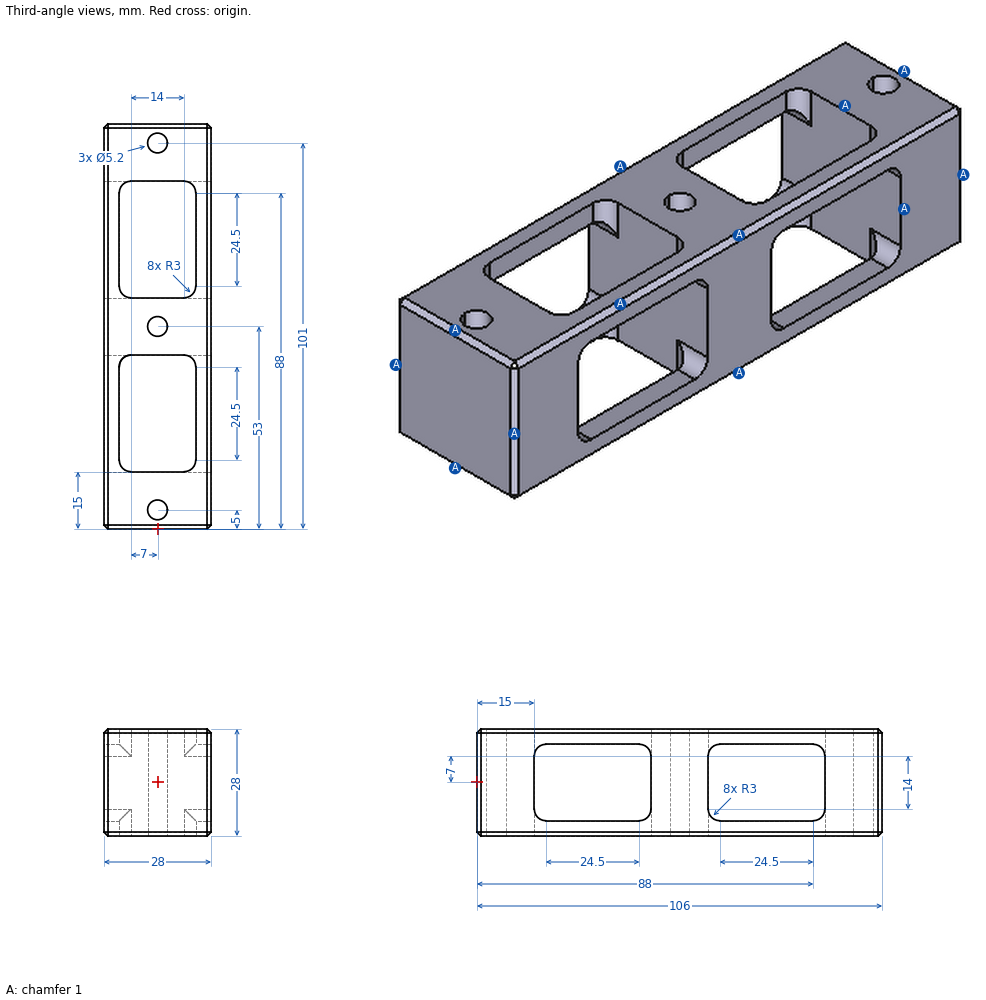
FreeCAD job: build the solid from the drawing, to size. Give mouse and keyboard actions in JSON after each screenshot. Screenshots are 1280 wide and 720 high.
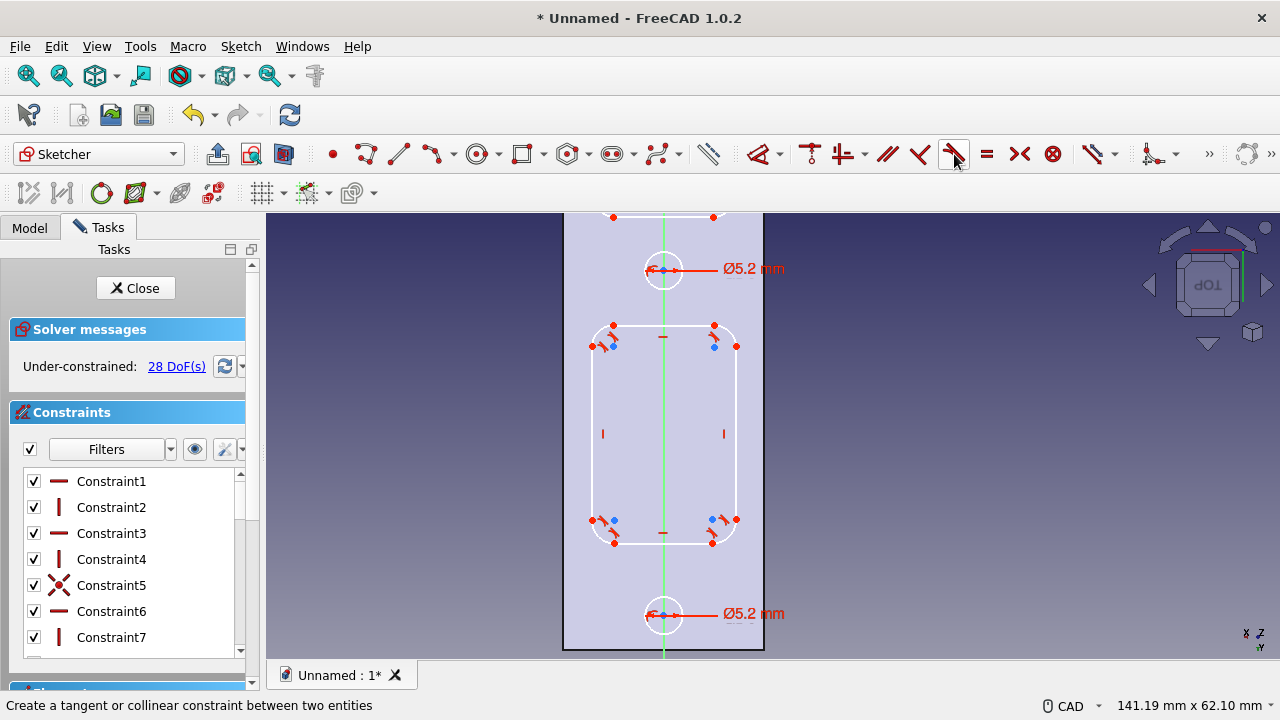
{"action": "left_click", "coordinate": [736, 468]}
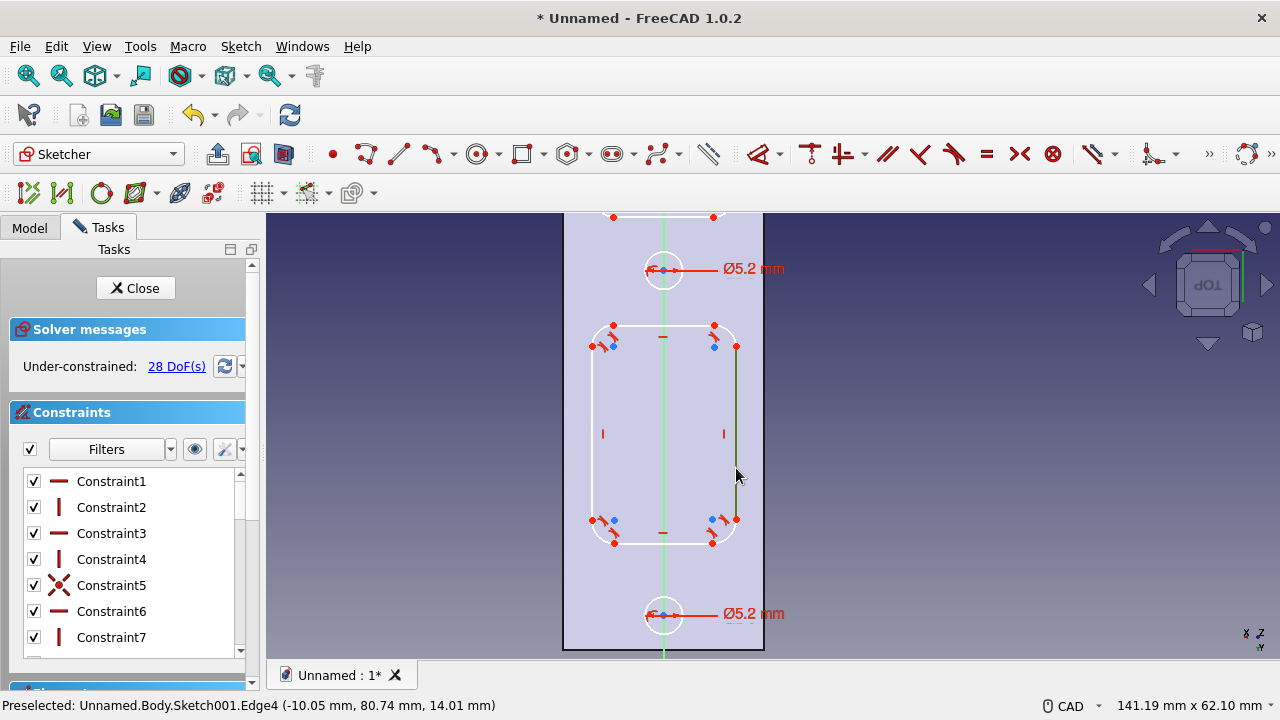
{"action": "scroll", "coordinate": [734, 337], "scroll_direction": "up", "scroll_amount": 2}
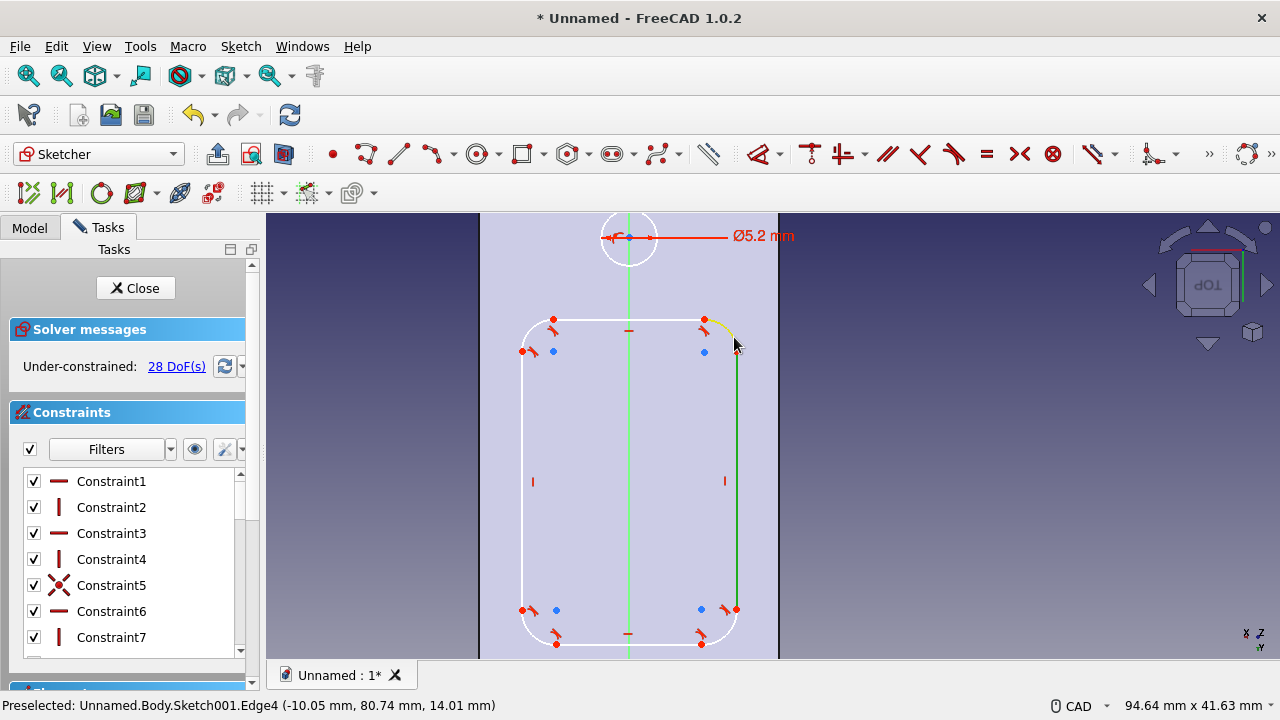
{"action": "left_click", "coordinate": [733, 337]}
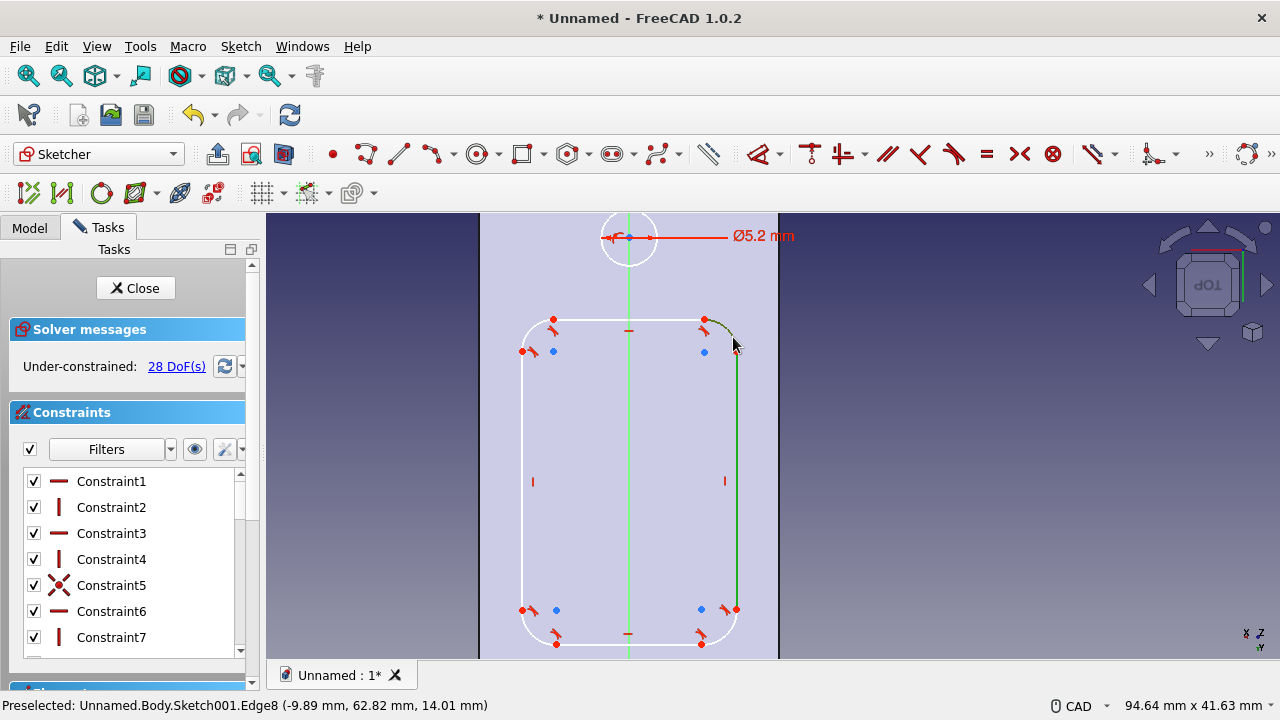
{"action": "left_click", "coordinate": [954, 154]}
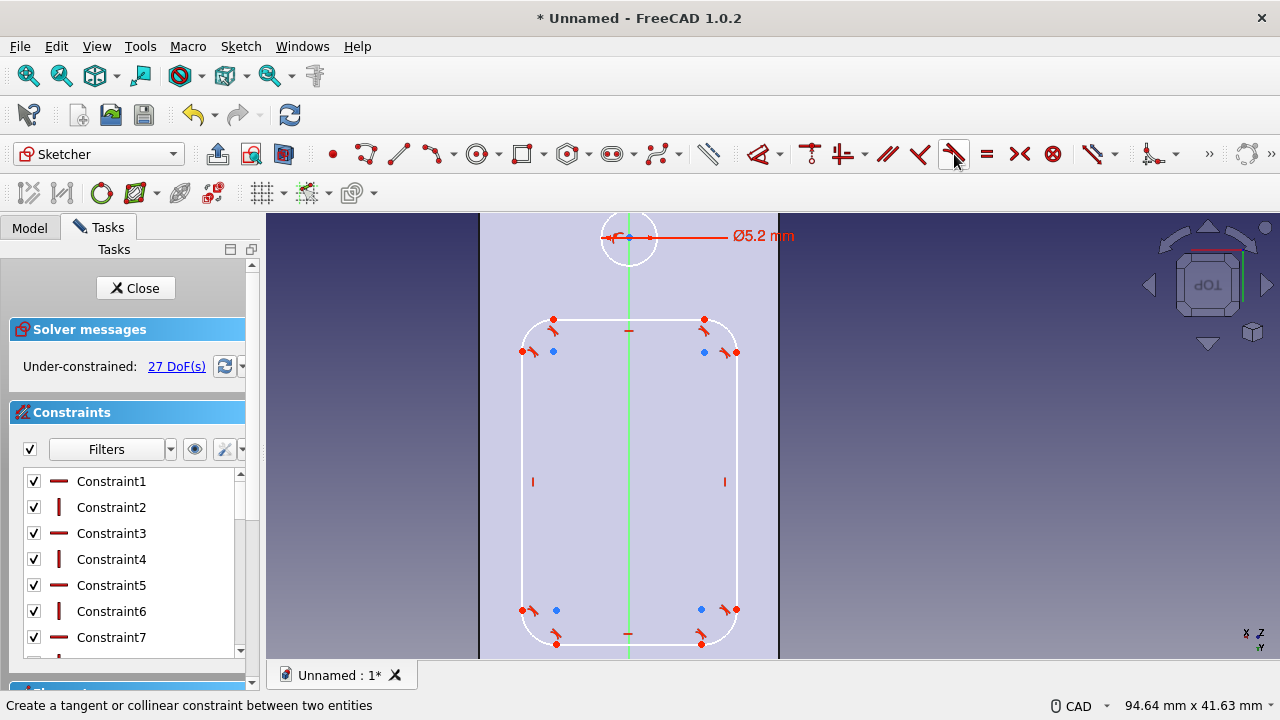
{"action": "scroll", "coordinate": [729, 505], "scroll_direction": "down", "scroll_amount": 7}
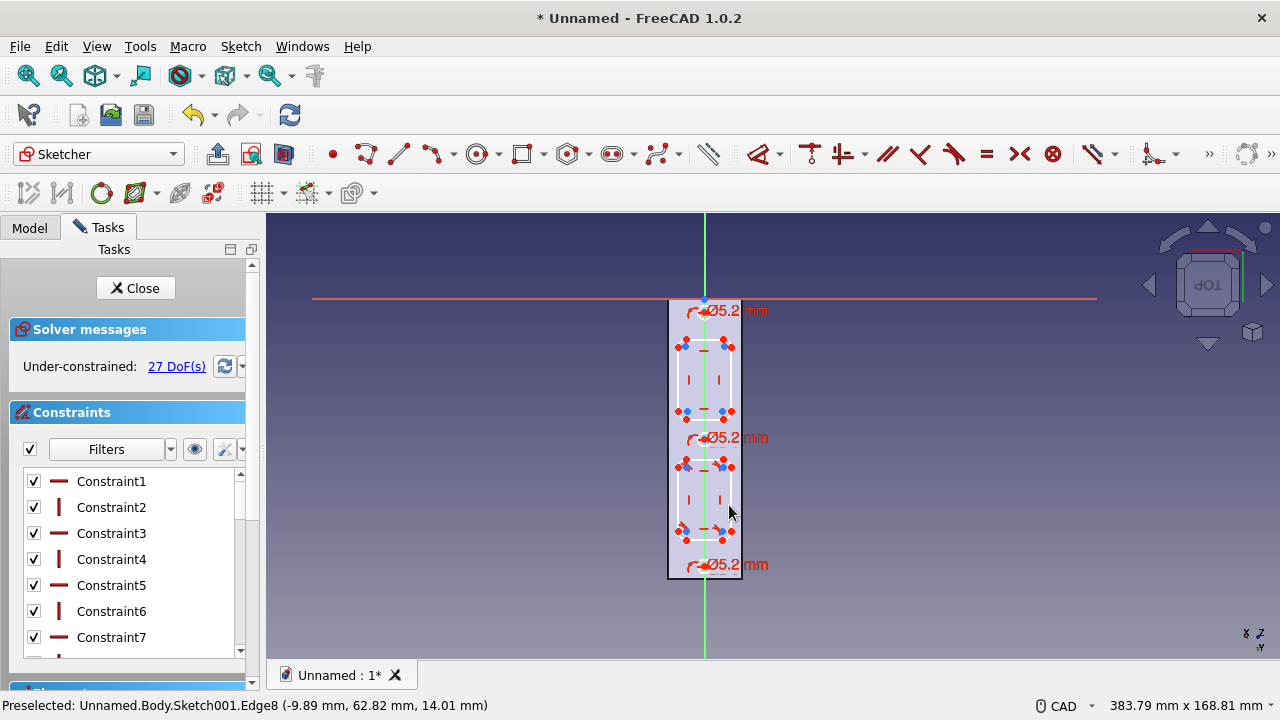
{"action": "scroll", "coordinate": [712, 340], "scroll_direction": "up", "scroll_amount": 4}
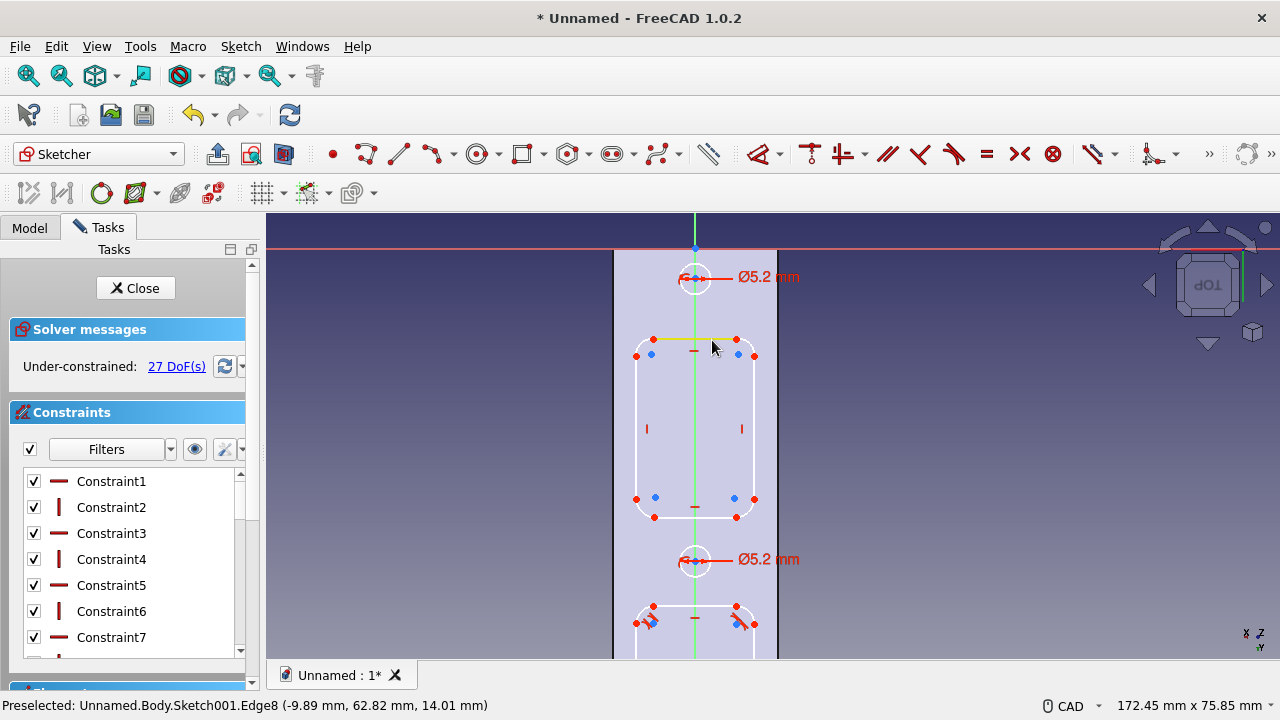
{"action": "left_click", "coordinate": [711, 339]}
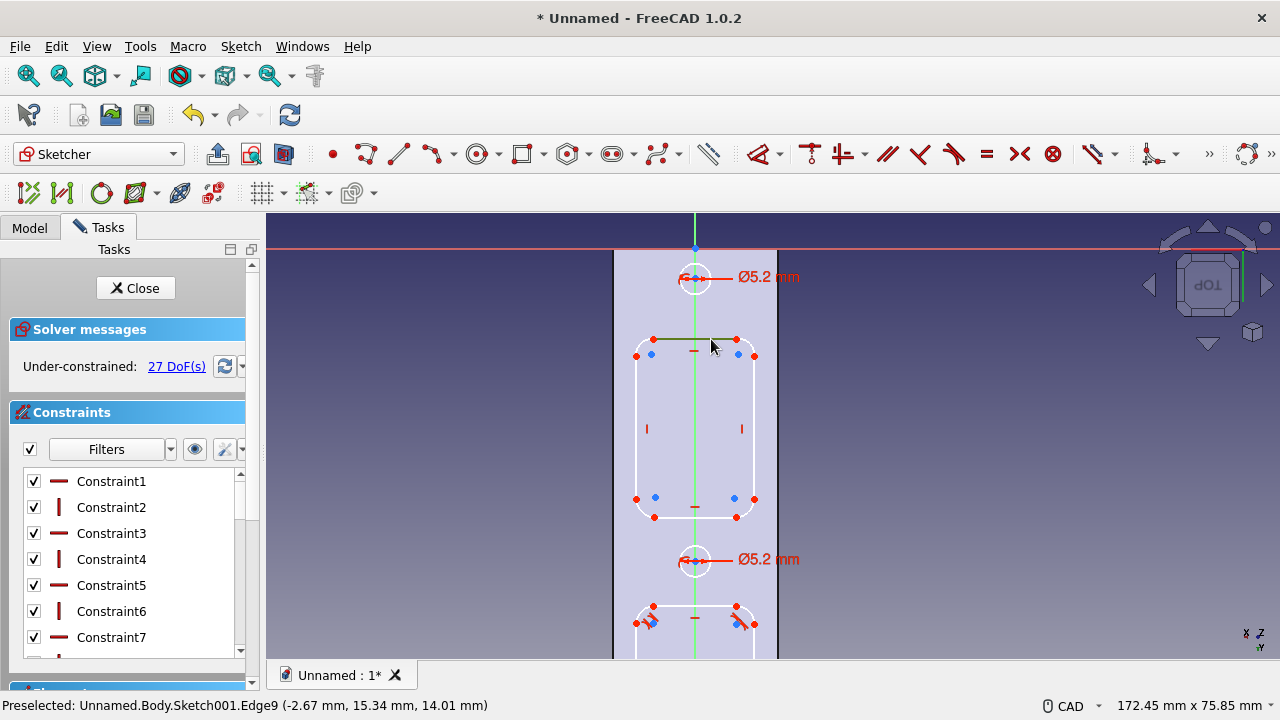
{"action": "left_click", "coordinate": [641, 344]}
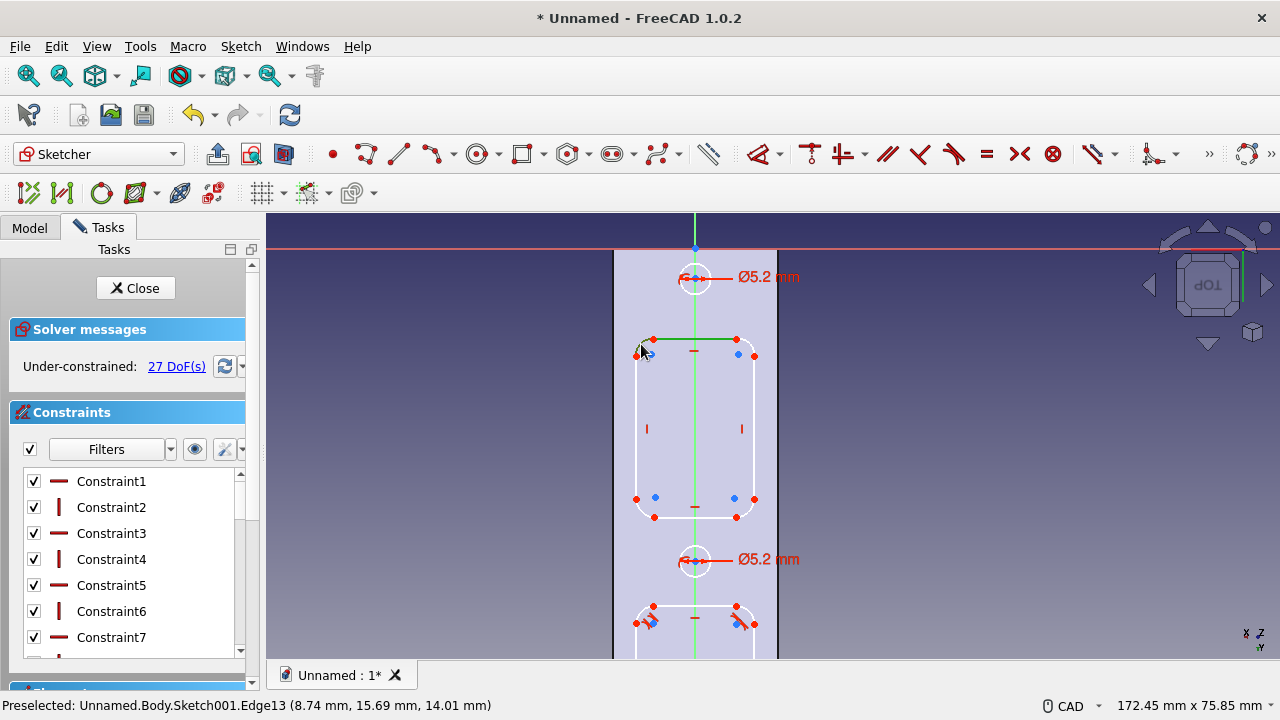
{"action": "left_click", "coordinate": [954, 154]}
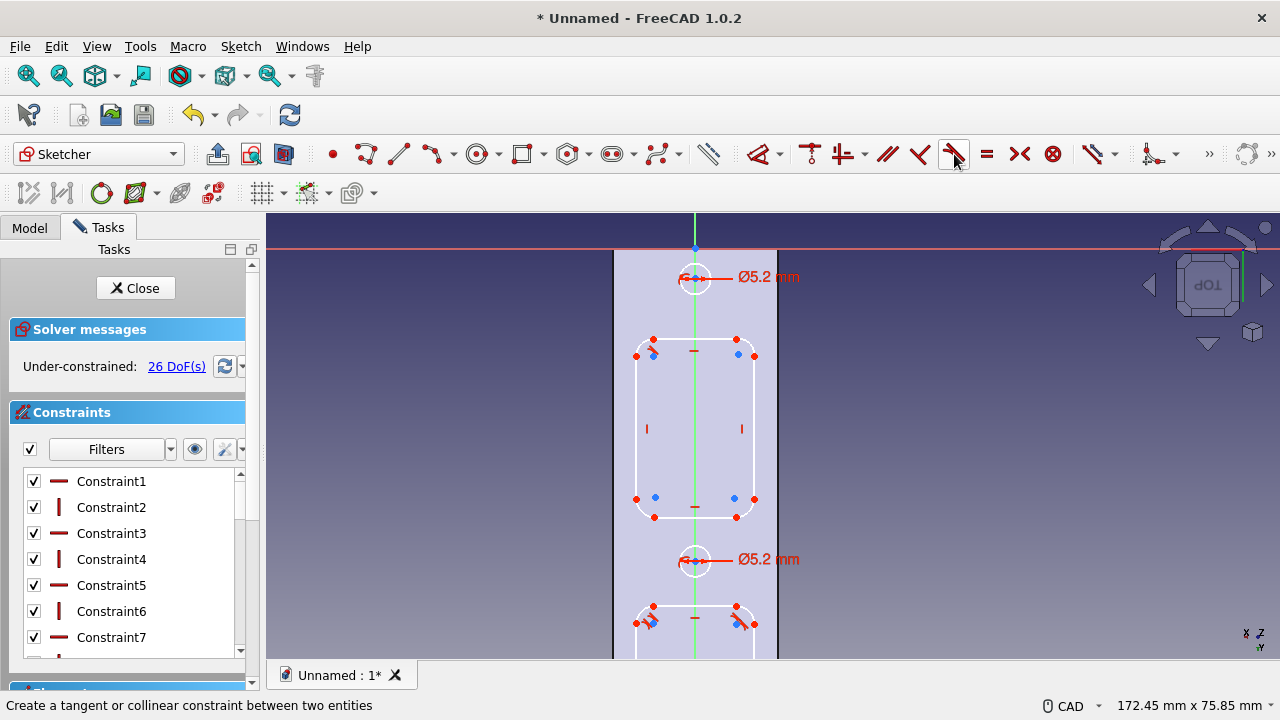
{"action": "left_click", "coordinate": [711, 339]}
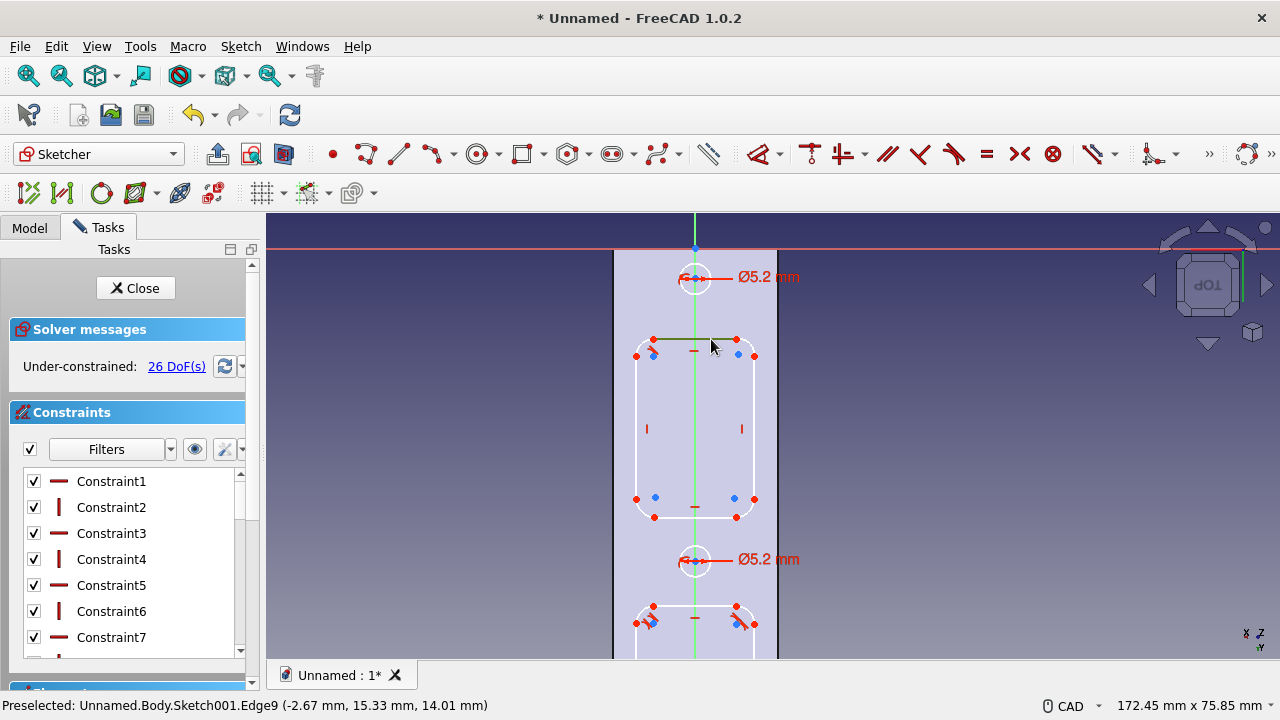
{"action": "left_click", "coordinate": [749, 343]}